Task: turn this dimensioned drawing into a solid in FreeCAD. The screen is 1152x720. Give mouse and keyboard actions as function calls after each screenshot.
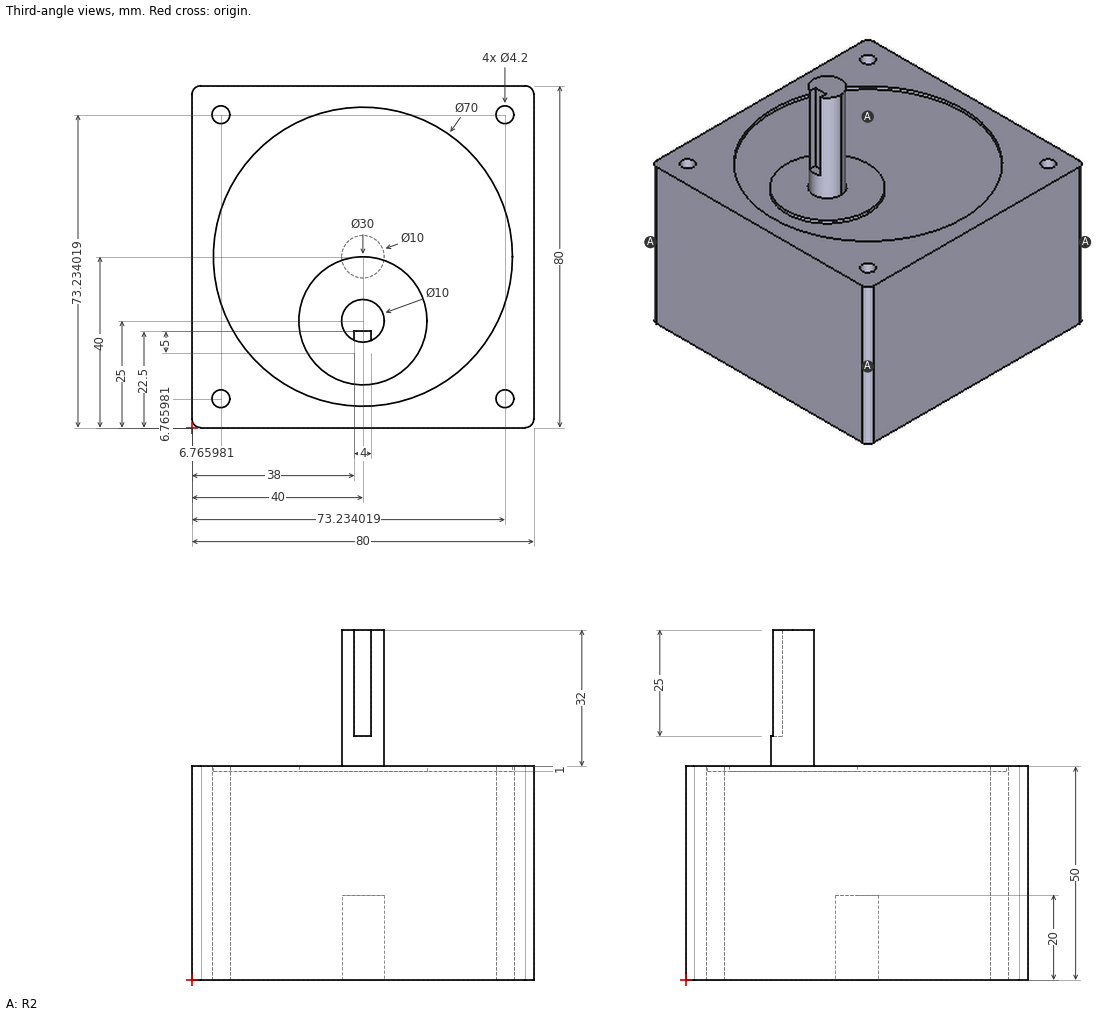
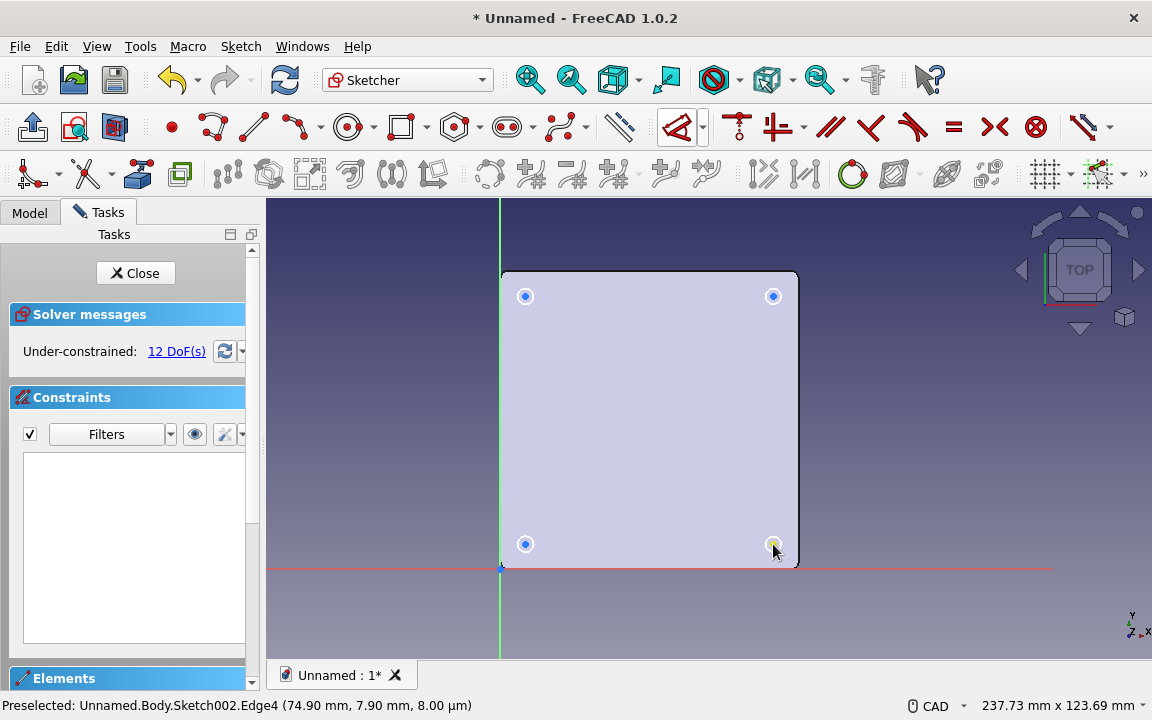
scroll(779, 291, up, 3)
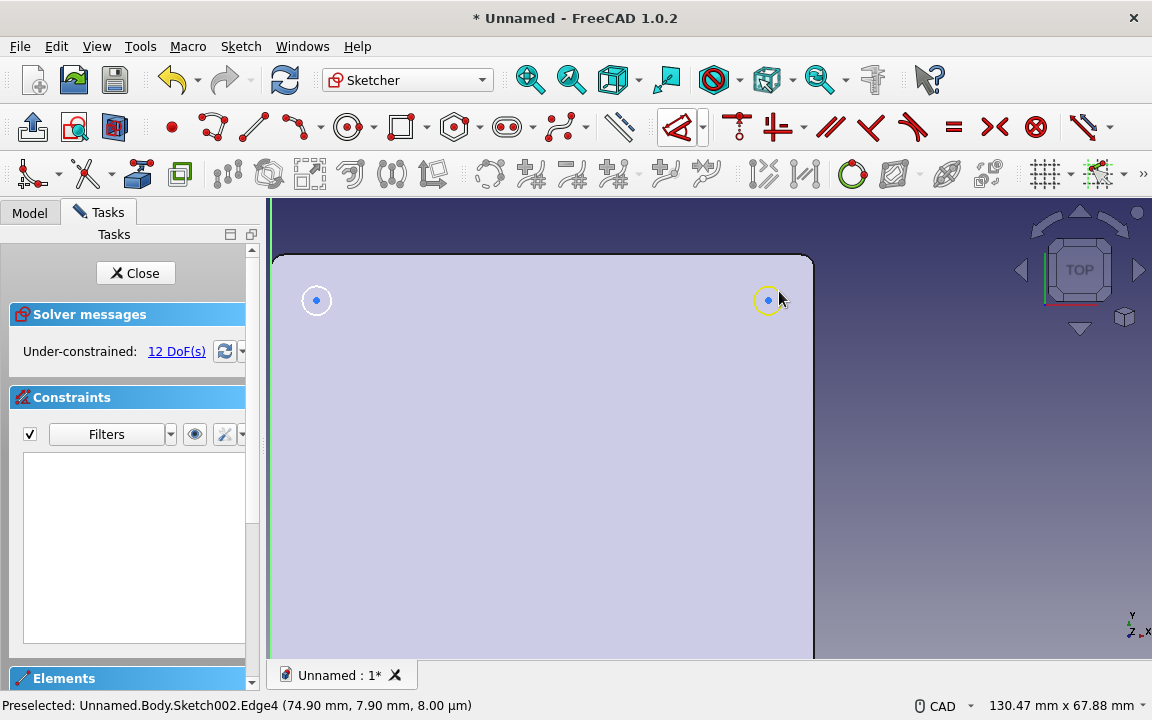
click(778, 291)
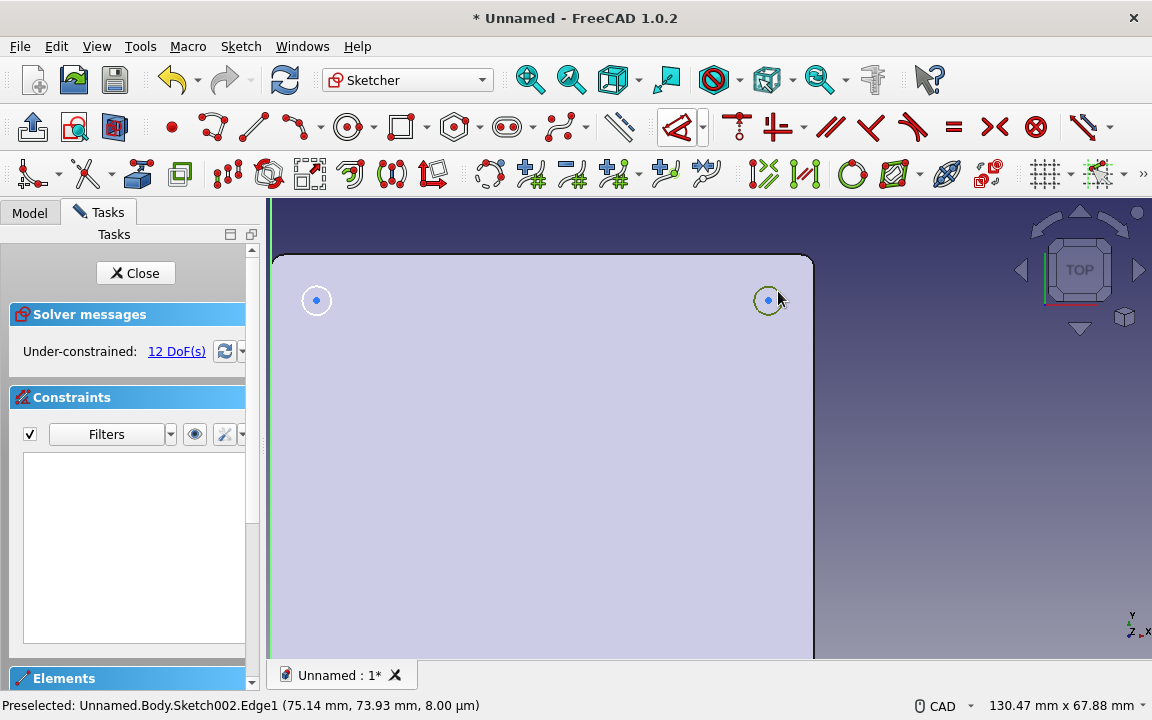
click(327, 291)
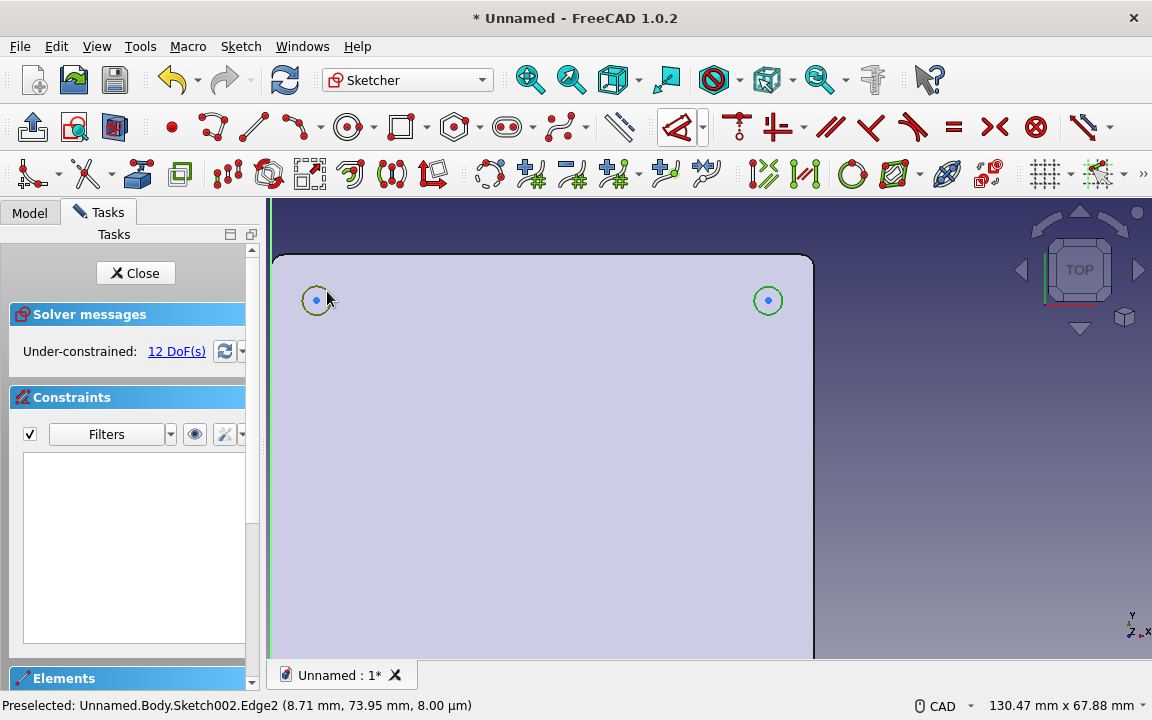
scroll(779, 291, down, 3)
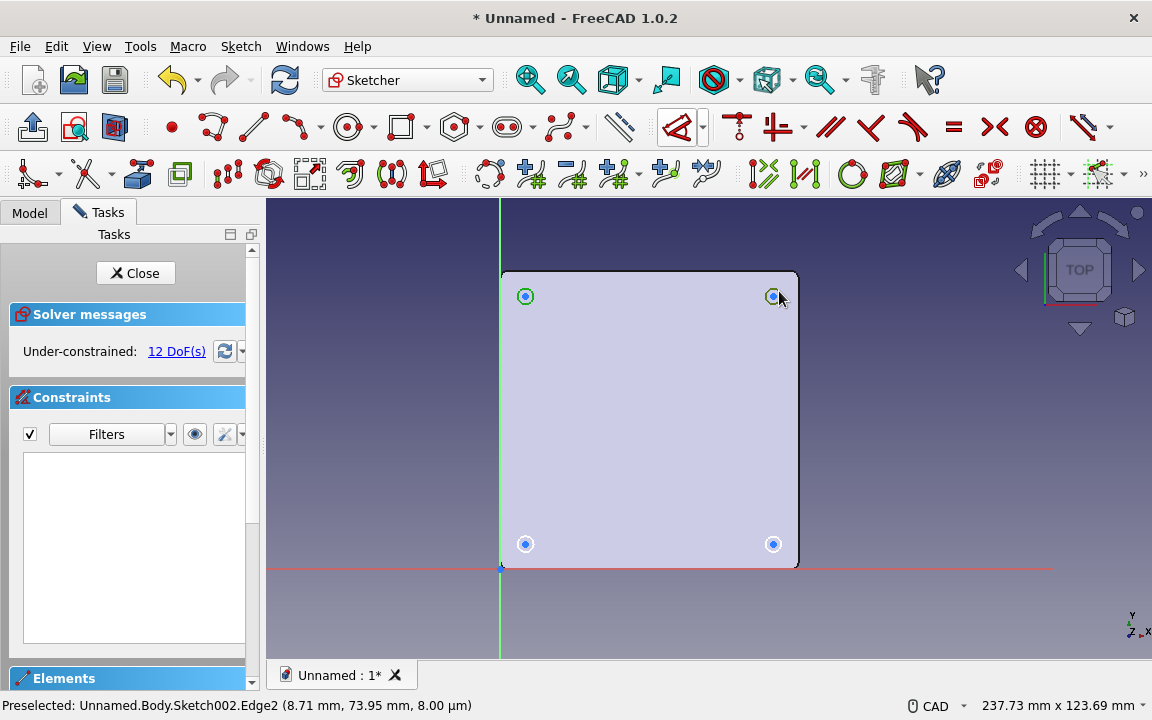
scroll(531, 539, up, 3)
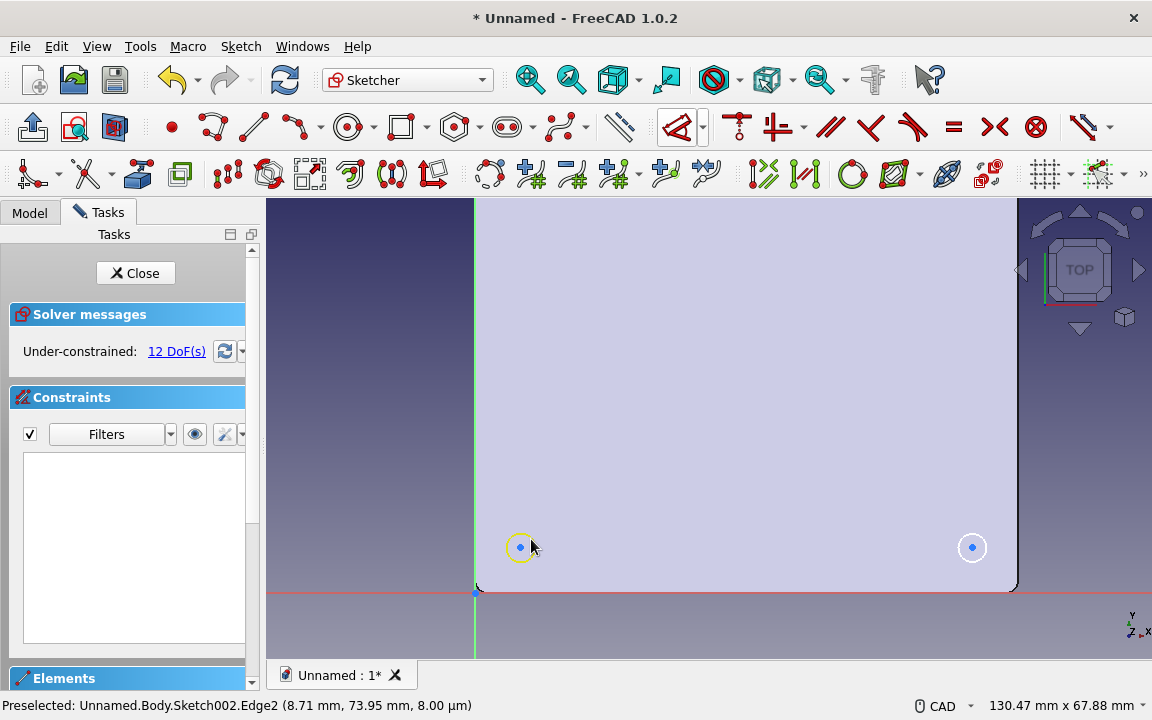
click(531, 538)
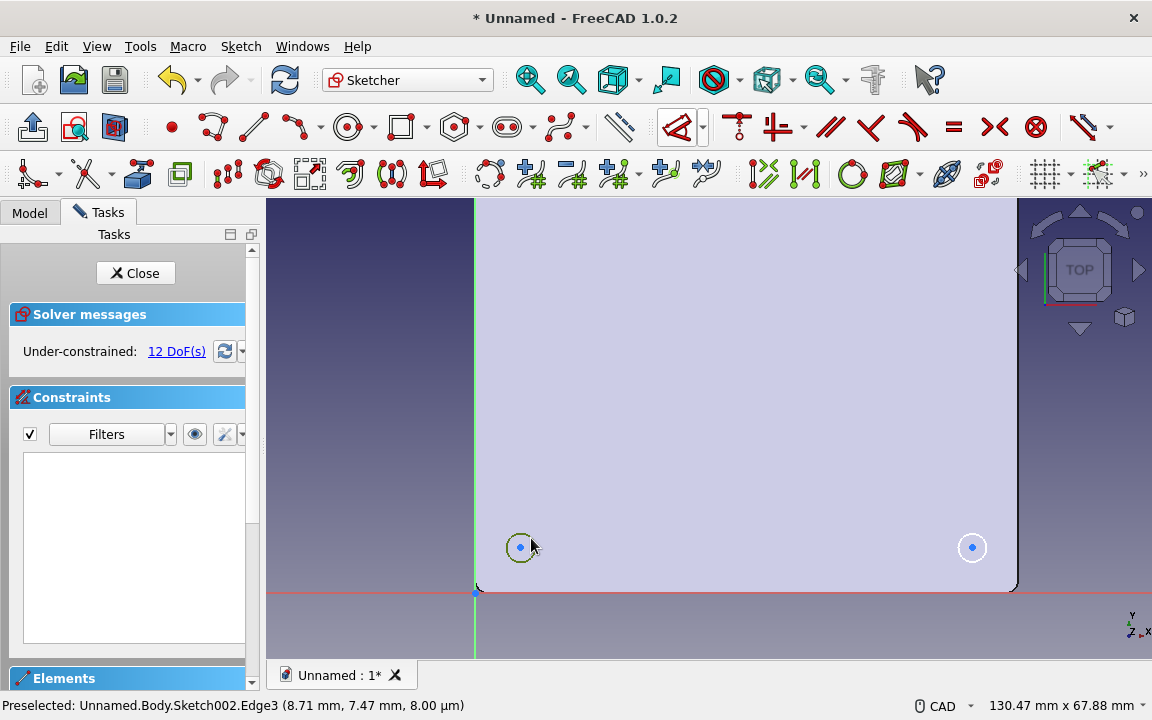
click(982, 538)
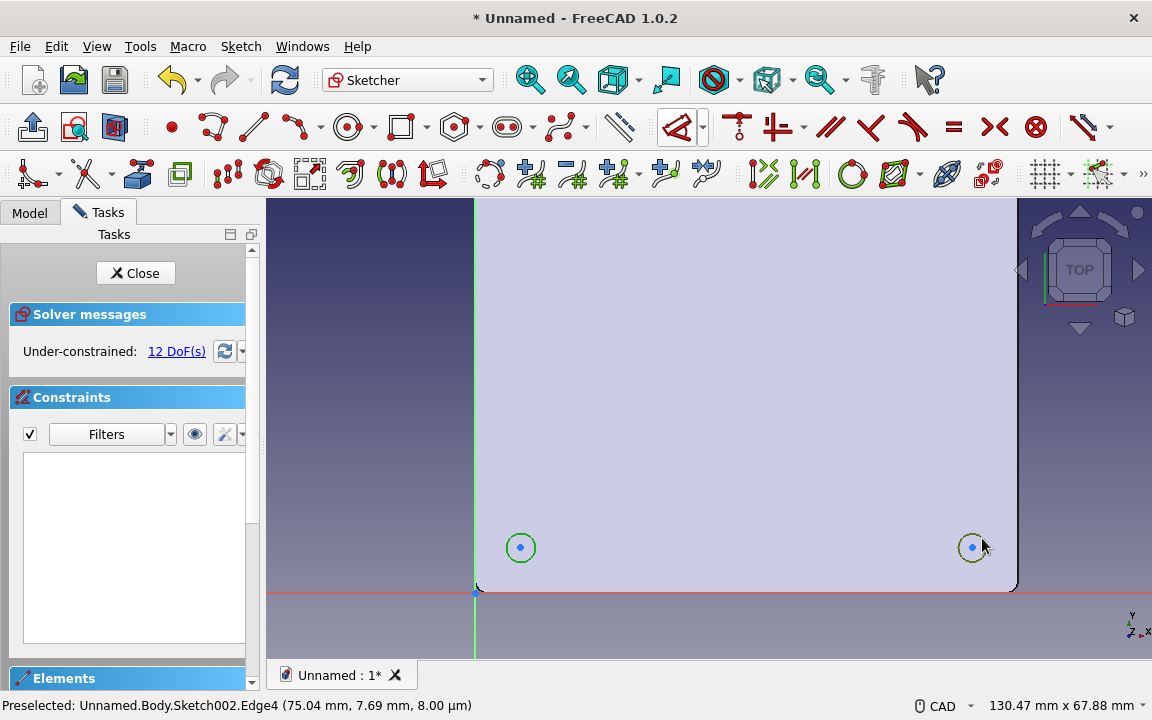
click(954, 128)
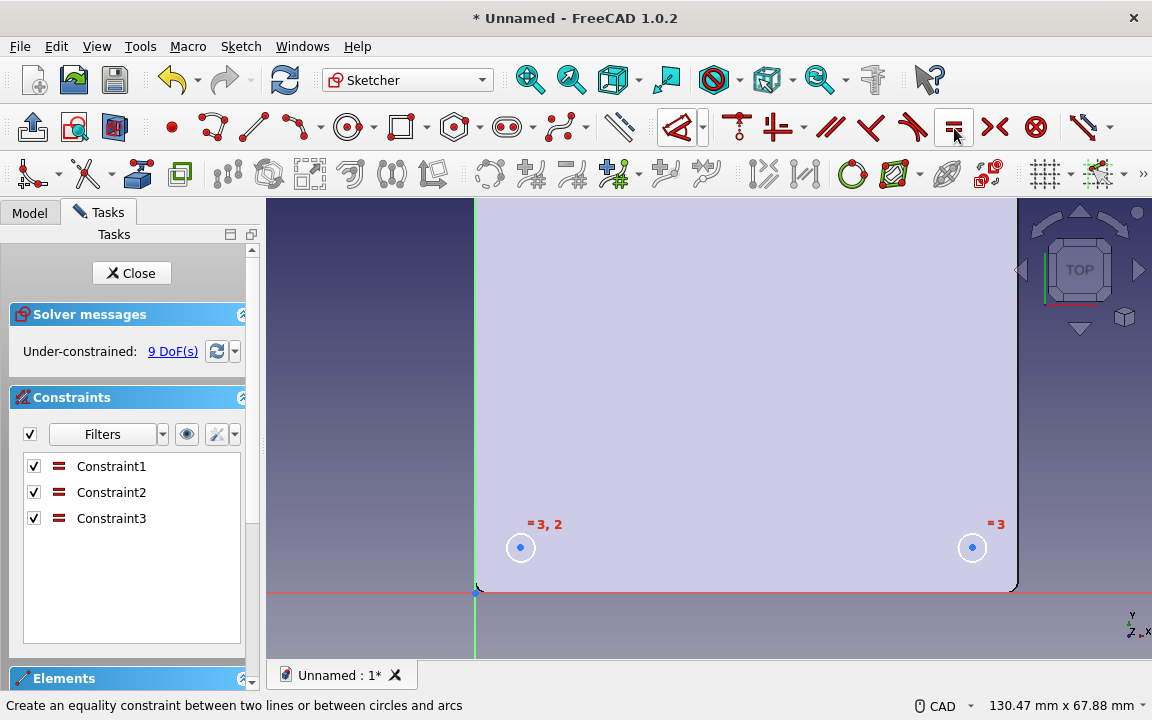
scroll(531, 539, down, 3)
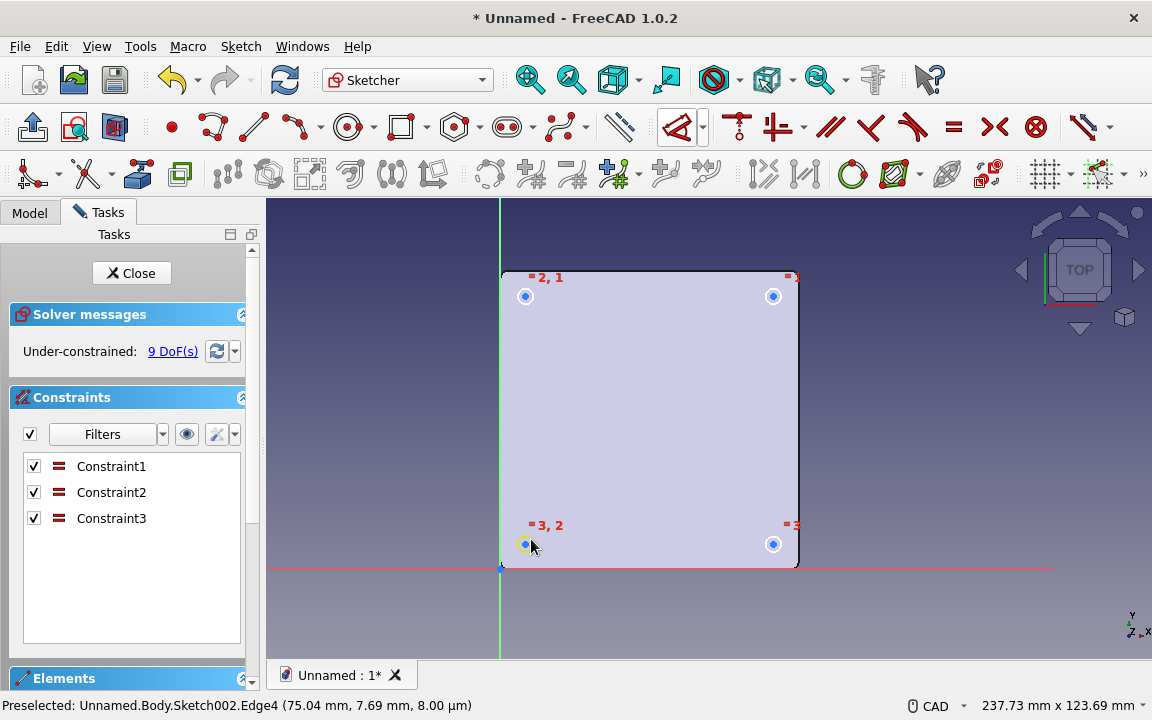
scroll(779, 291, up, 5)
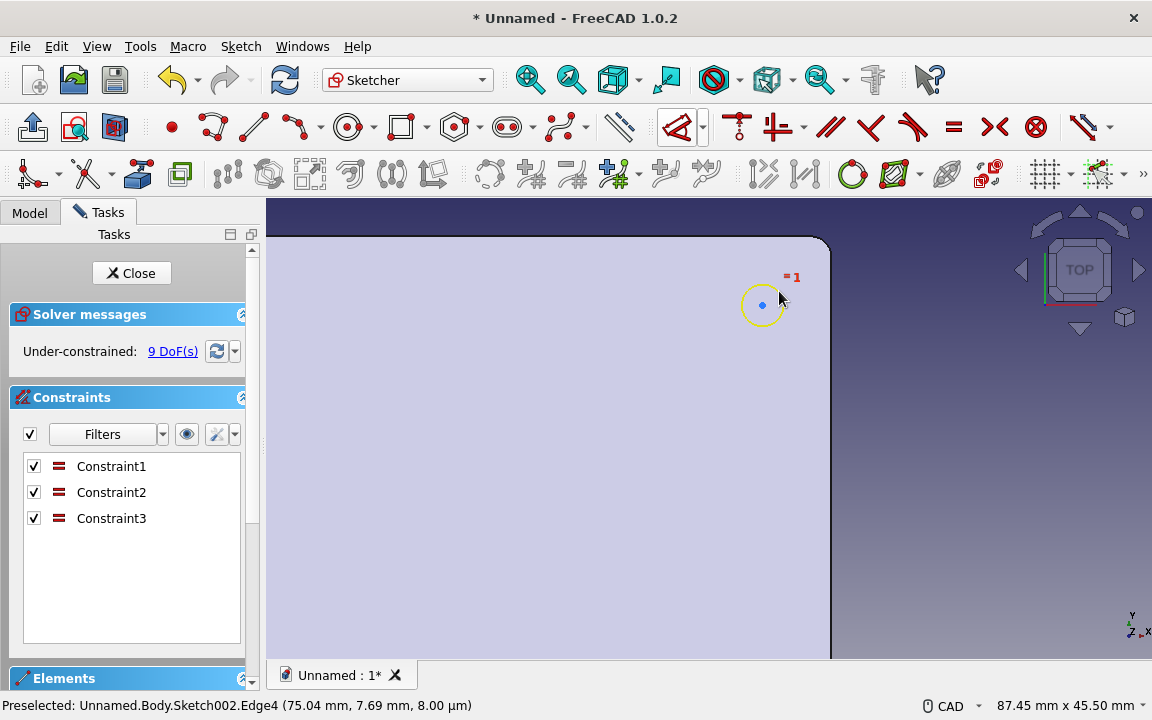
click(777, 291)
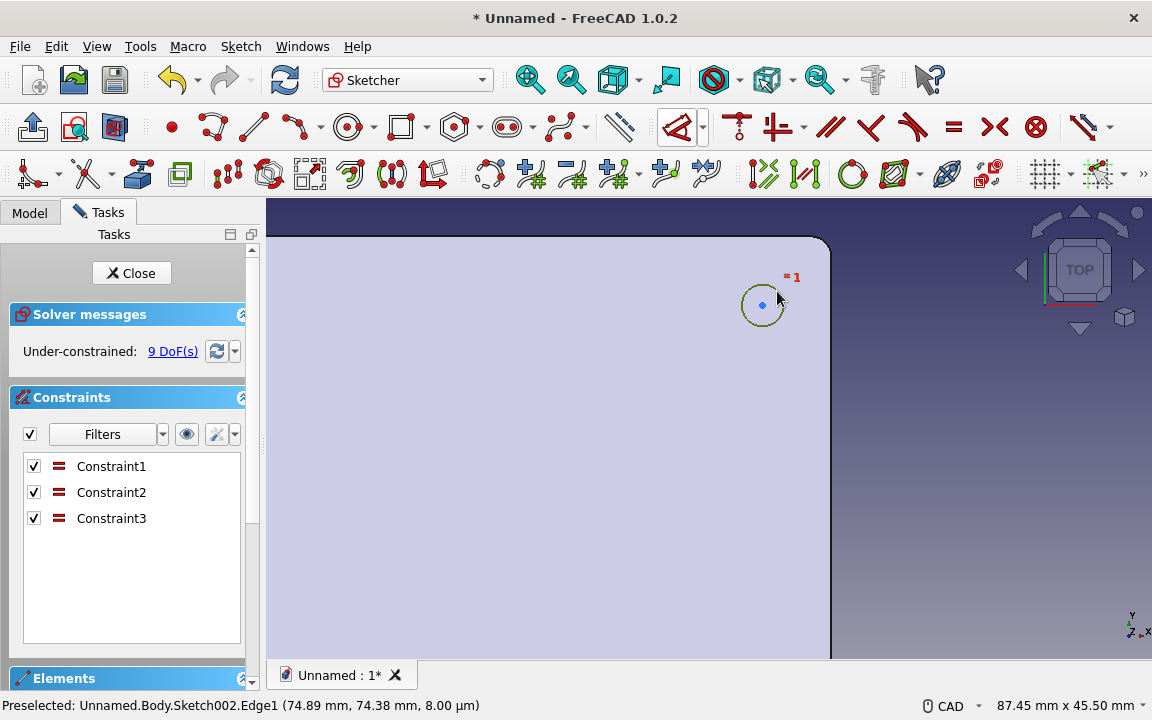
click(702, 128)